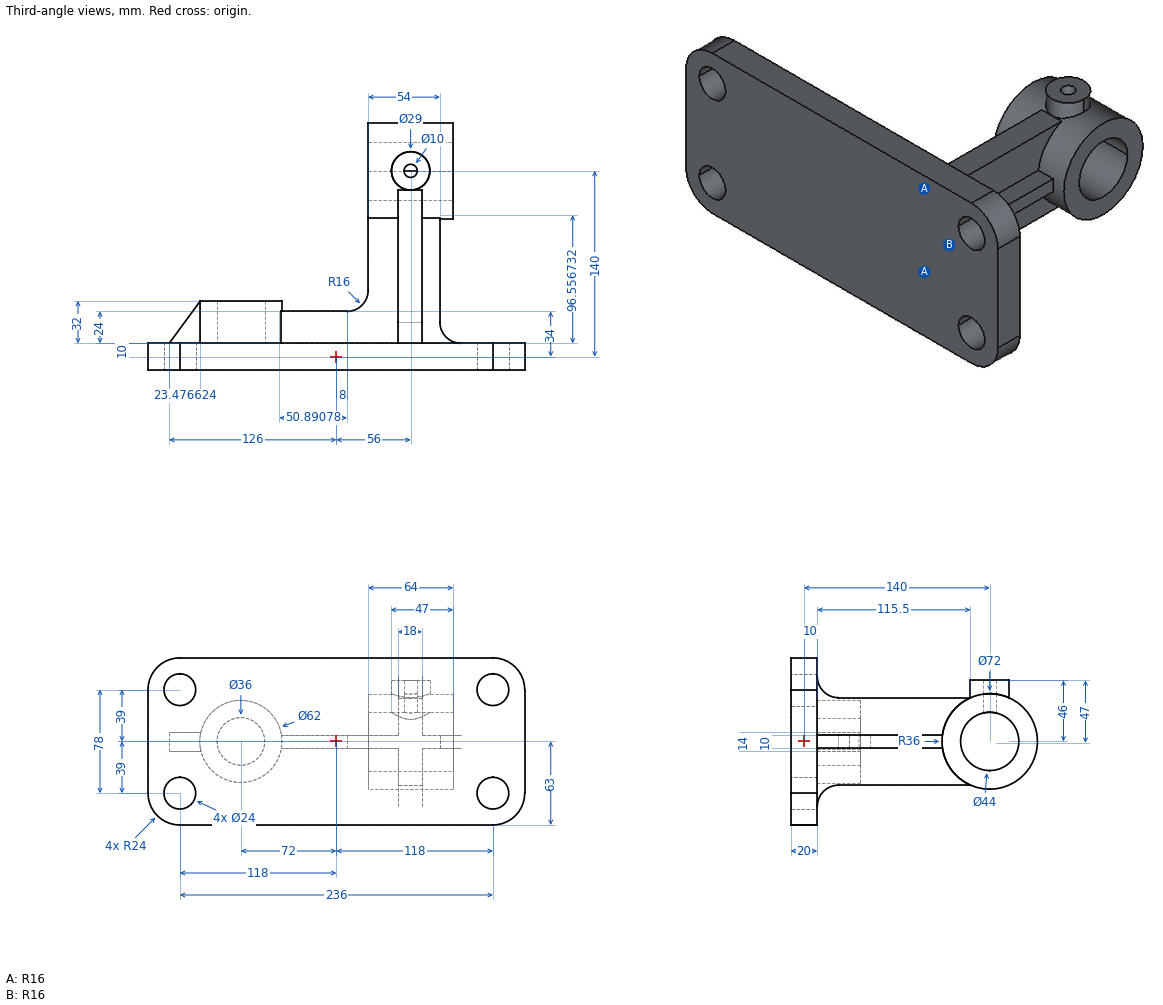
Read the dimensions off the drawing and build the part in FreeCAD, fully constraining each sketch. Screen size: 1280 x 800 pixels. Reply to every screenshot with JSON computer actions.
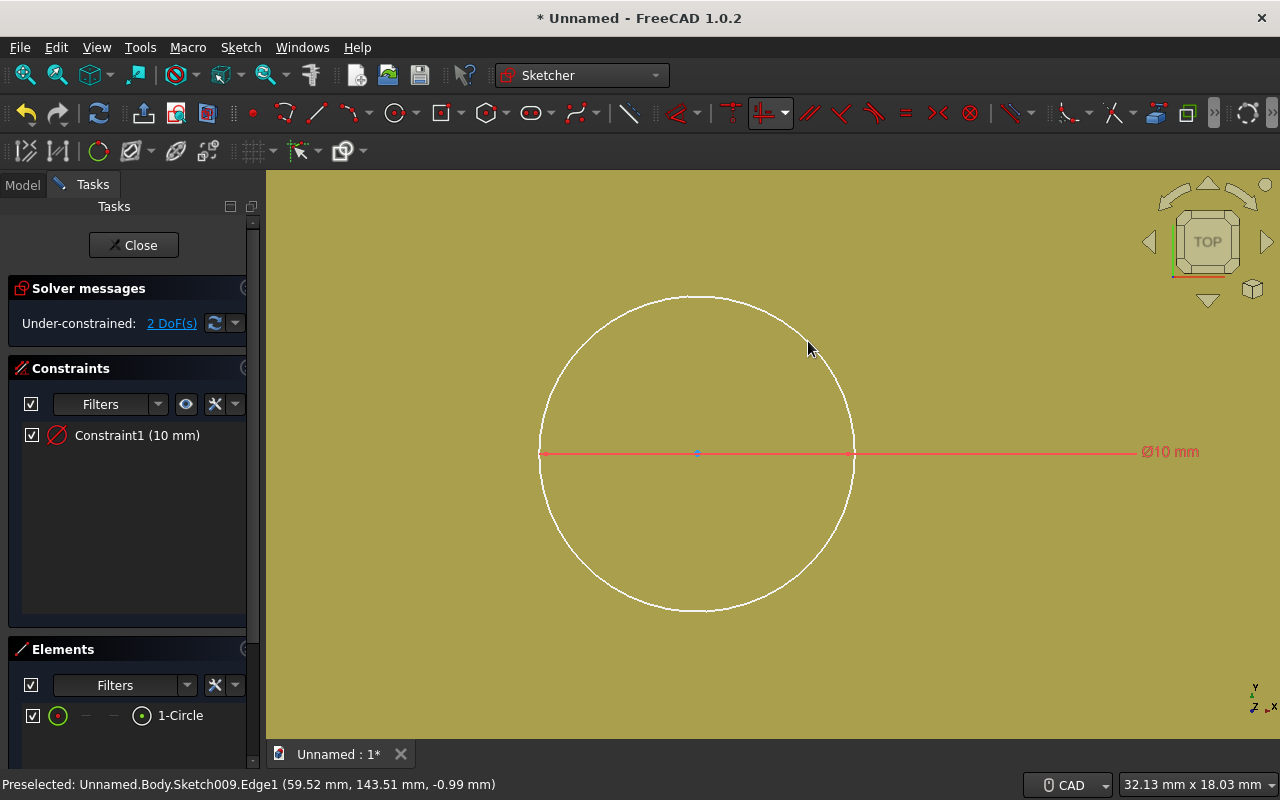
{"action": "left_click", "coordinate": [676, 114]}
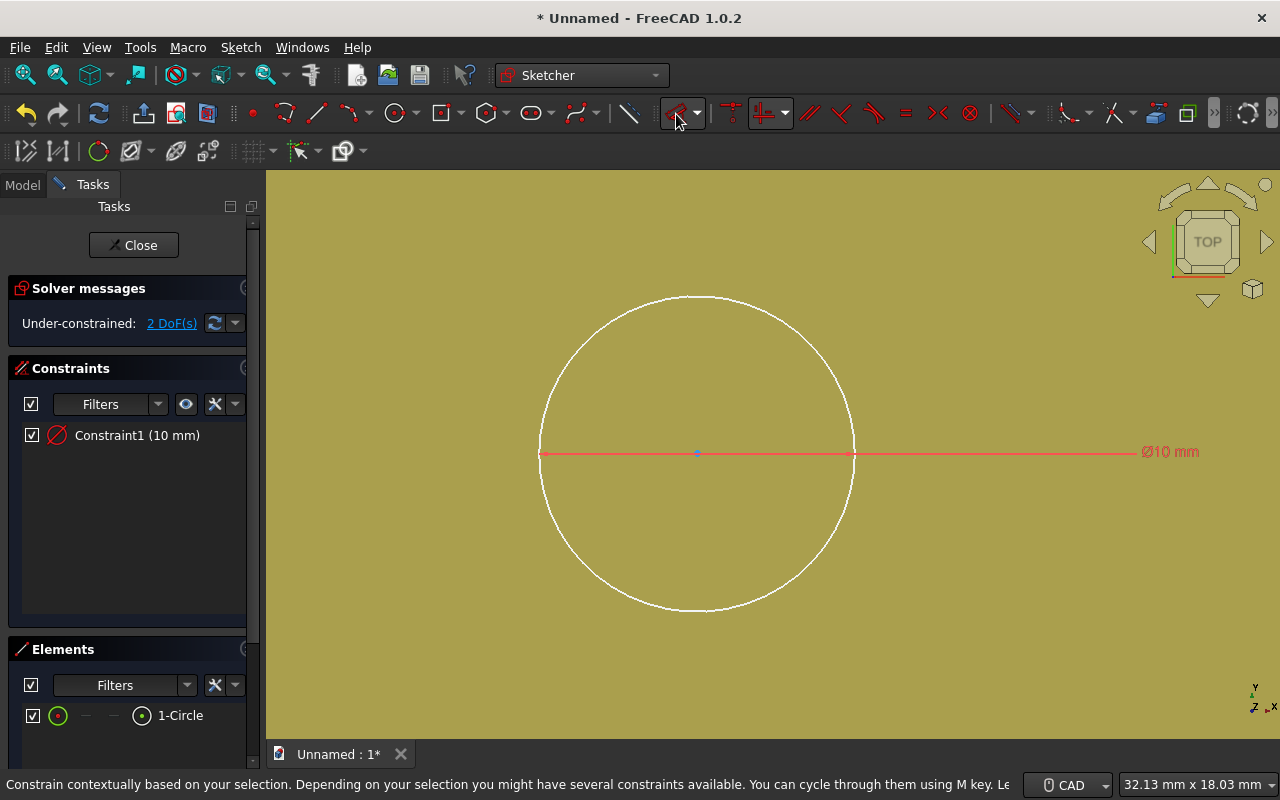
{"action": "left_click", "coordinate": [697, 454]}
{"action": "left_click", "coordinate": [496, 420]}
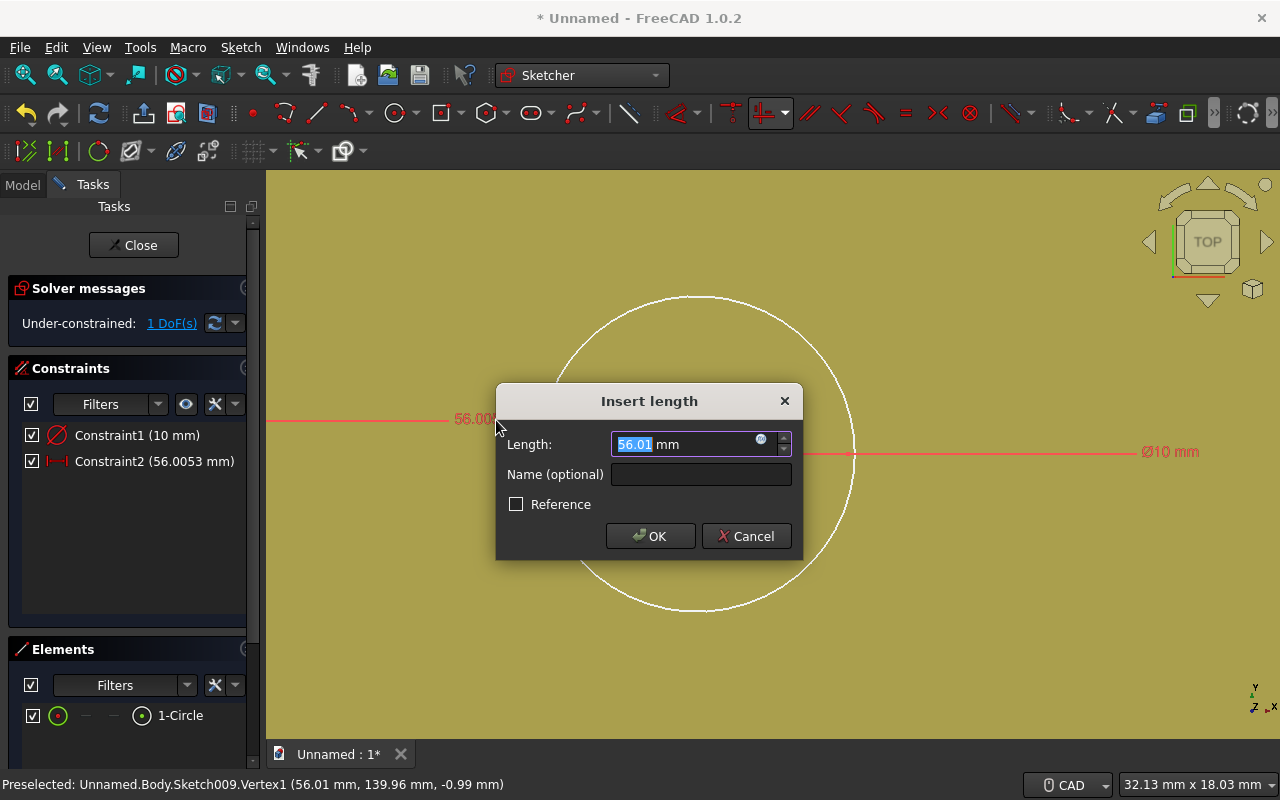
{"action": "type", "text": "56"}
{"action": "key", "text": "Return"}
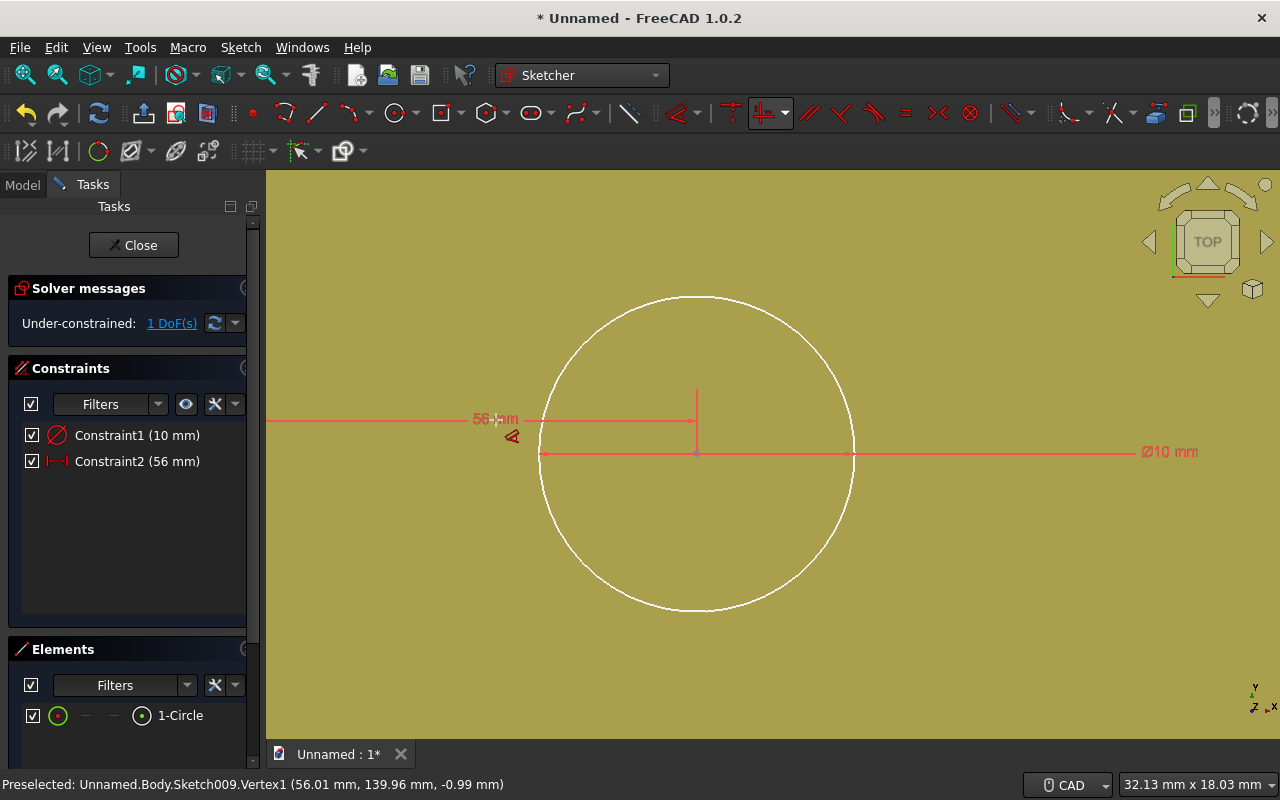
{"action": "left_click", "coordinate": [697, 454]}
{"action": "left_click", "coordinate": [731, 583]}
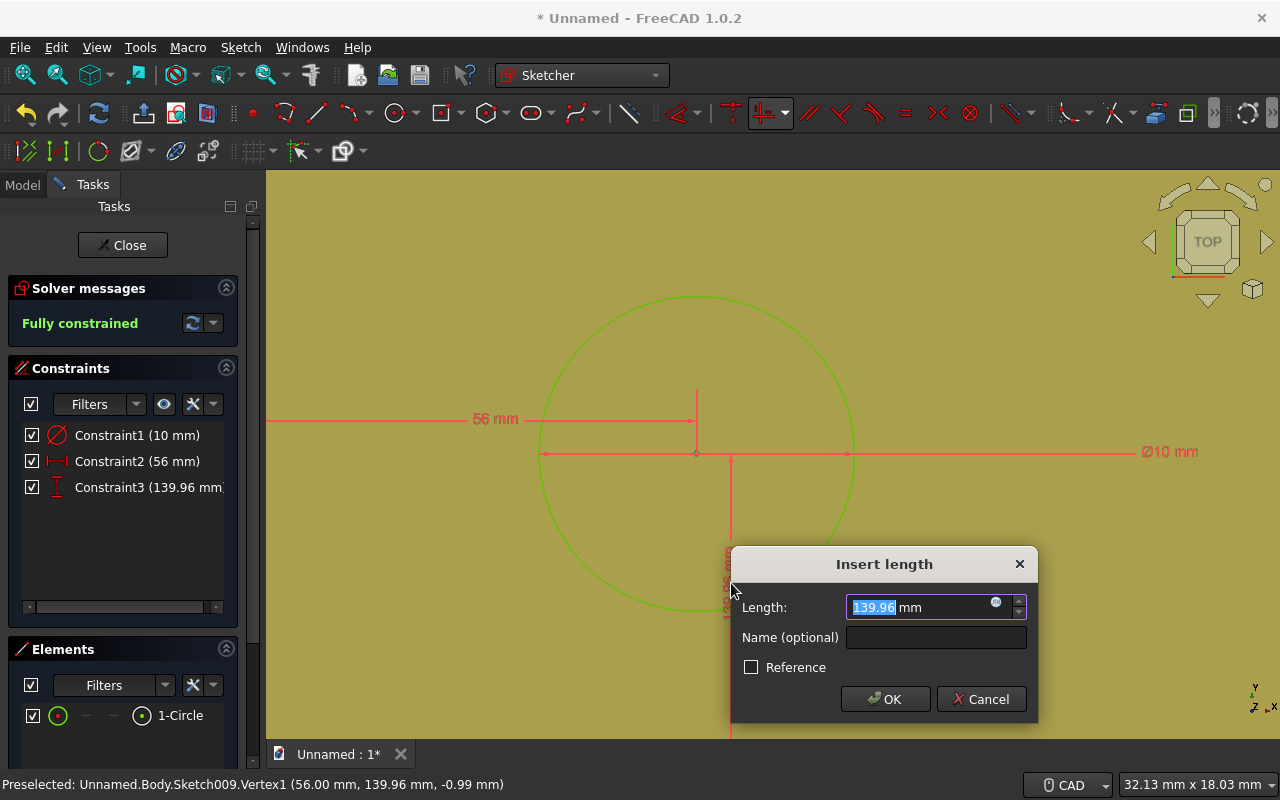
{"action": "type", "text": "140"}
{"action": "key", "text": "Return"}
{"action": "key", "text": "Escape"}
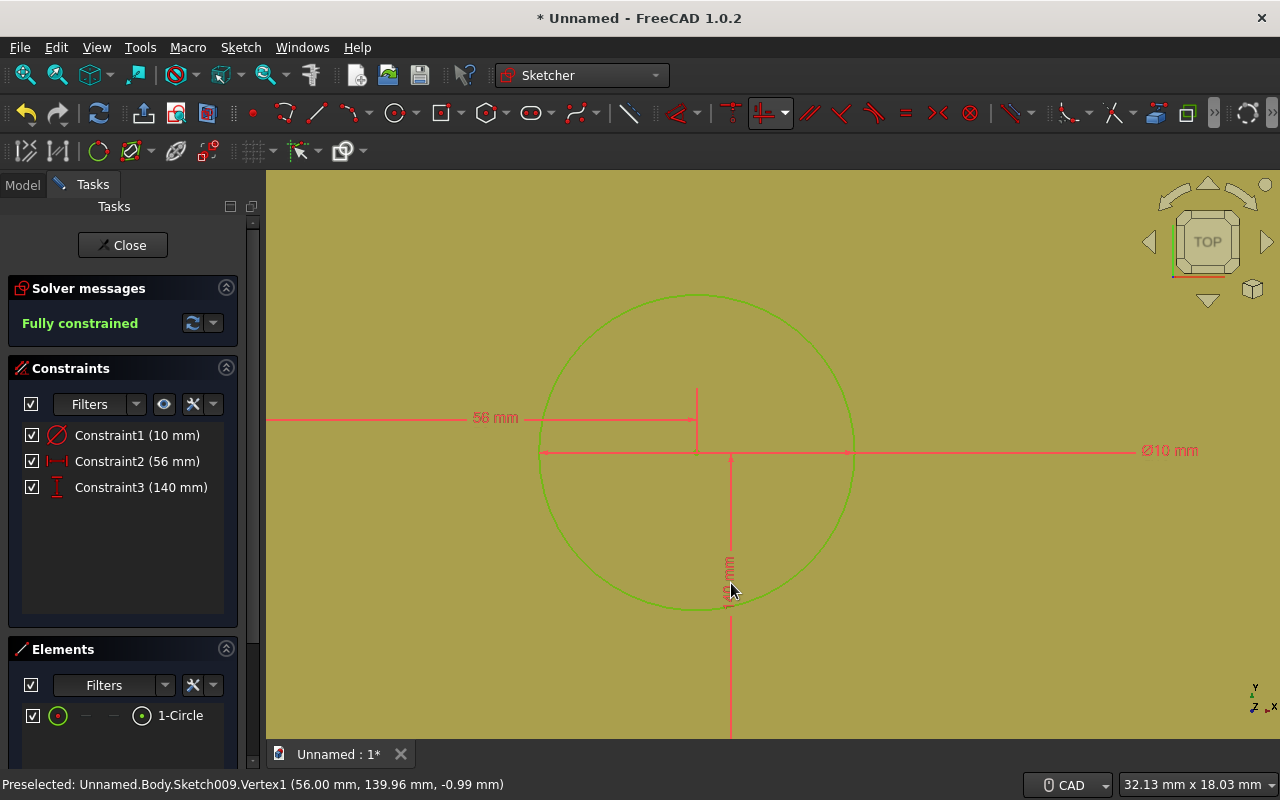
{"action": "left_click", "coordinate": [123, 245]}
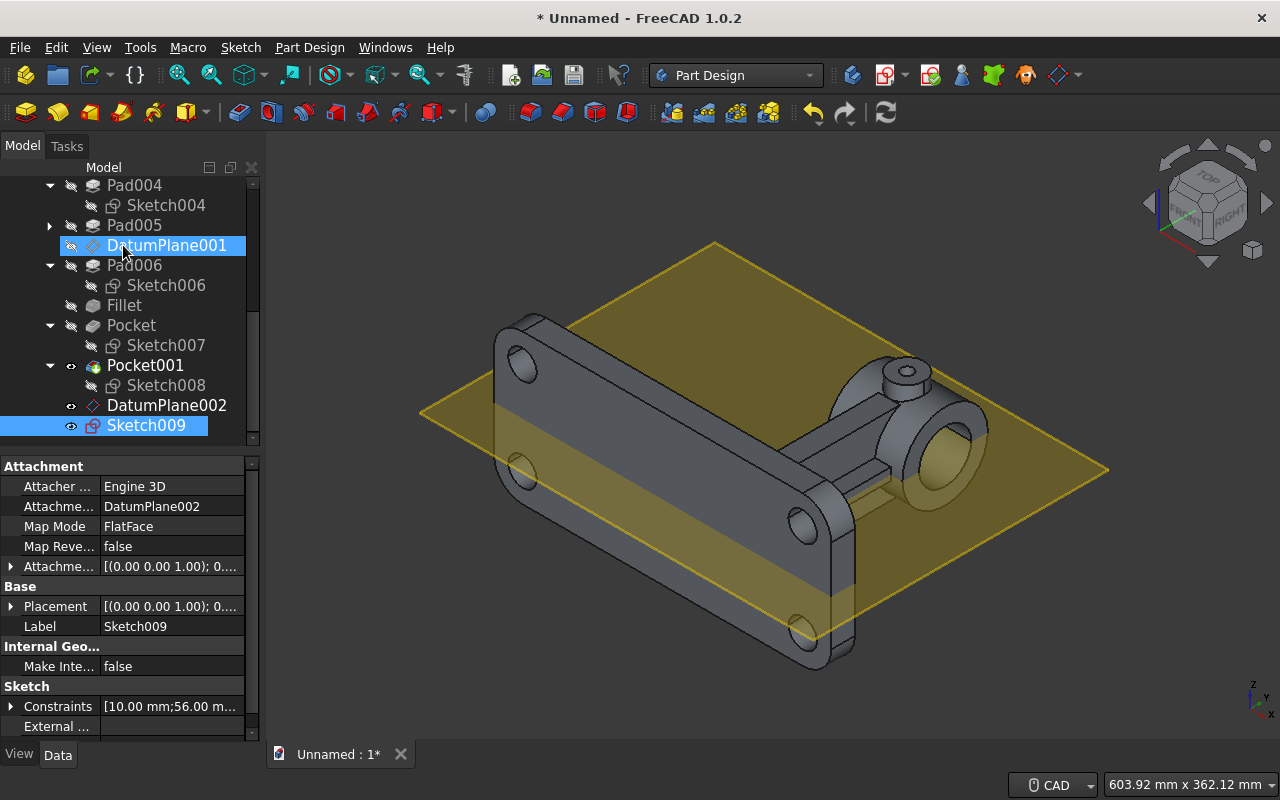
{"action": "left_click", "coordinate": [240, 112]}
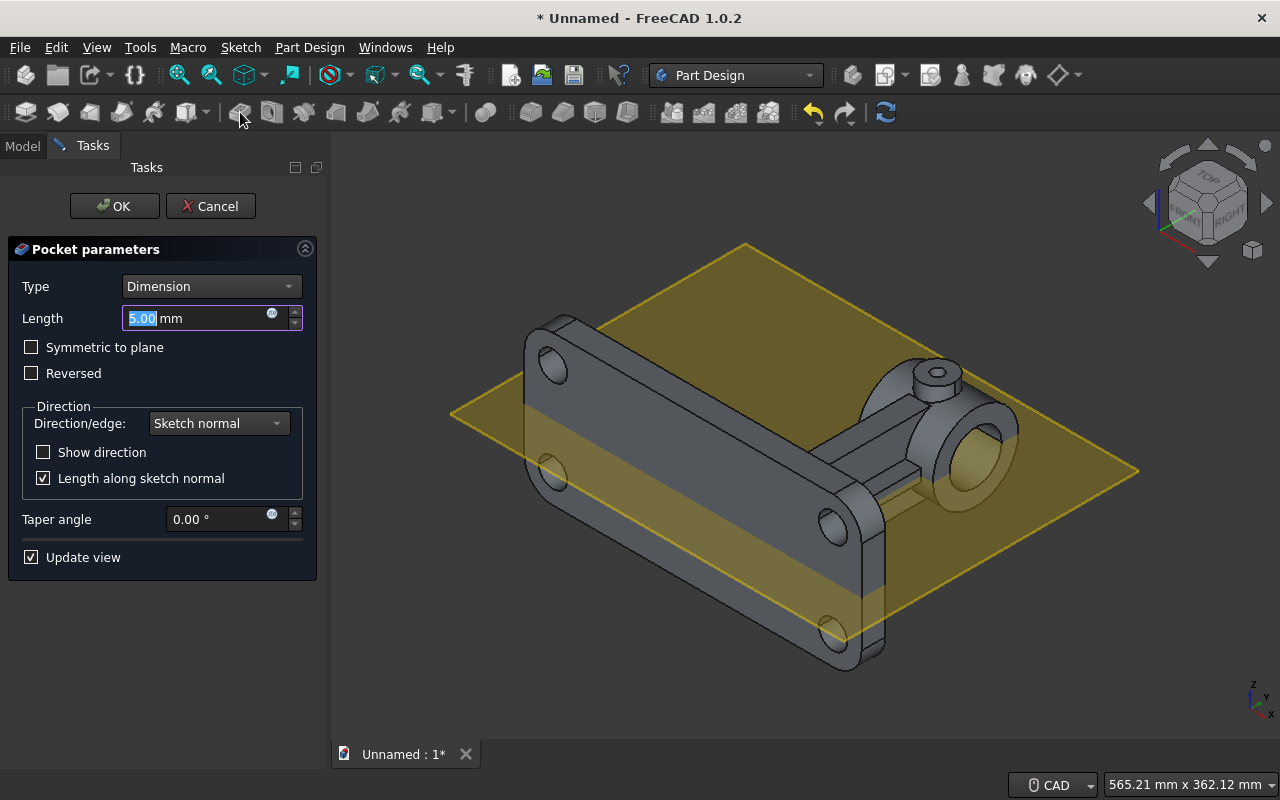
{"action": "type", "text": "47"}
{"action": "key", "text": "Tab"}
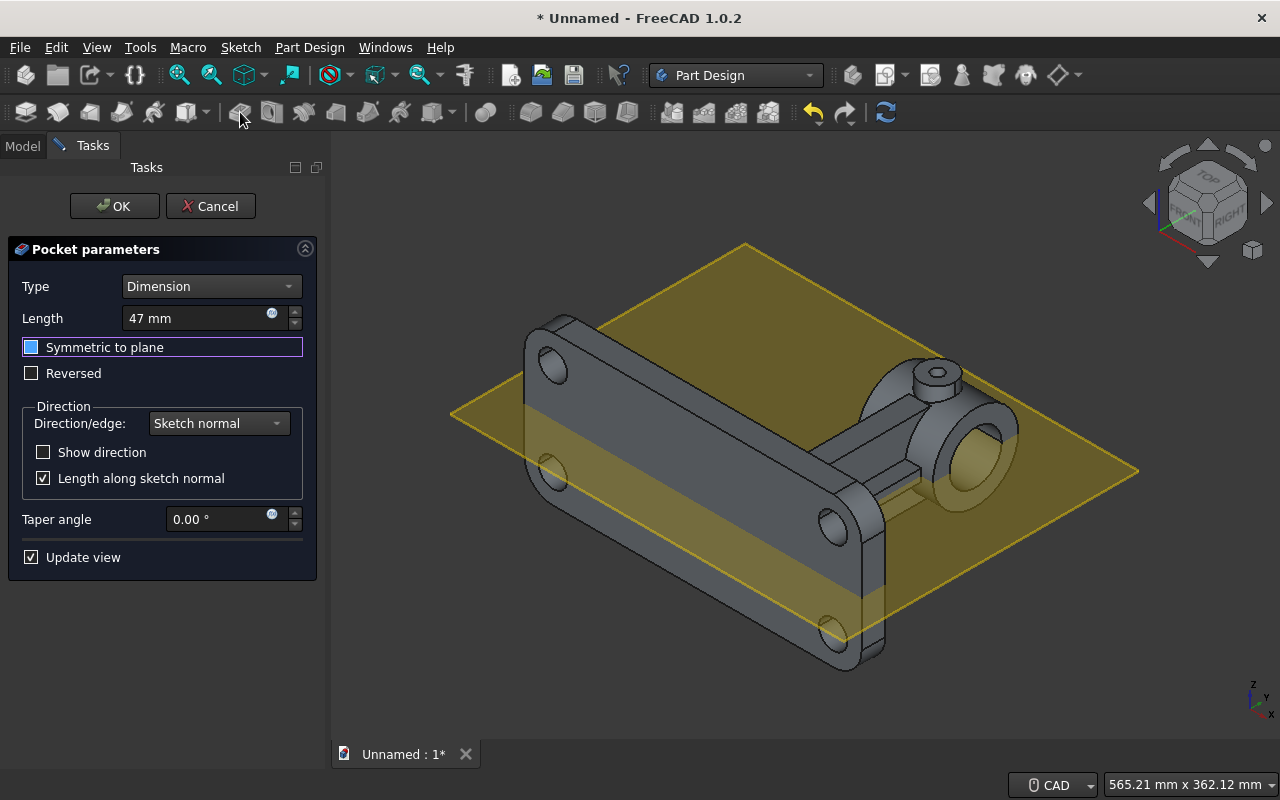
{"action": "left_click", "coordinate": [30, 373]}